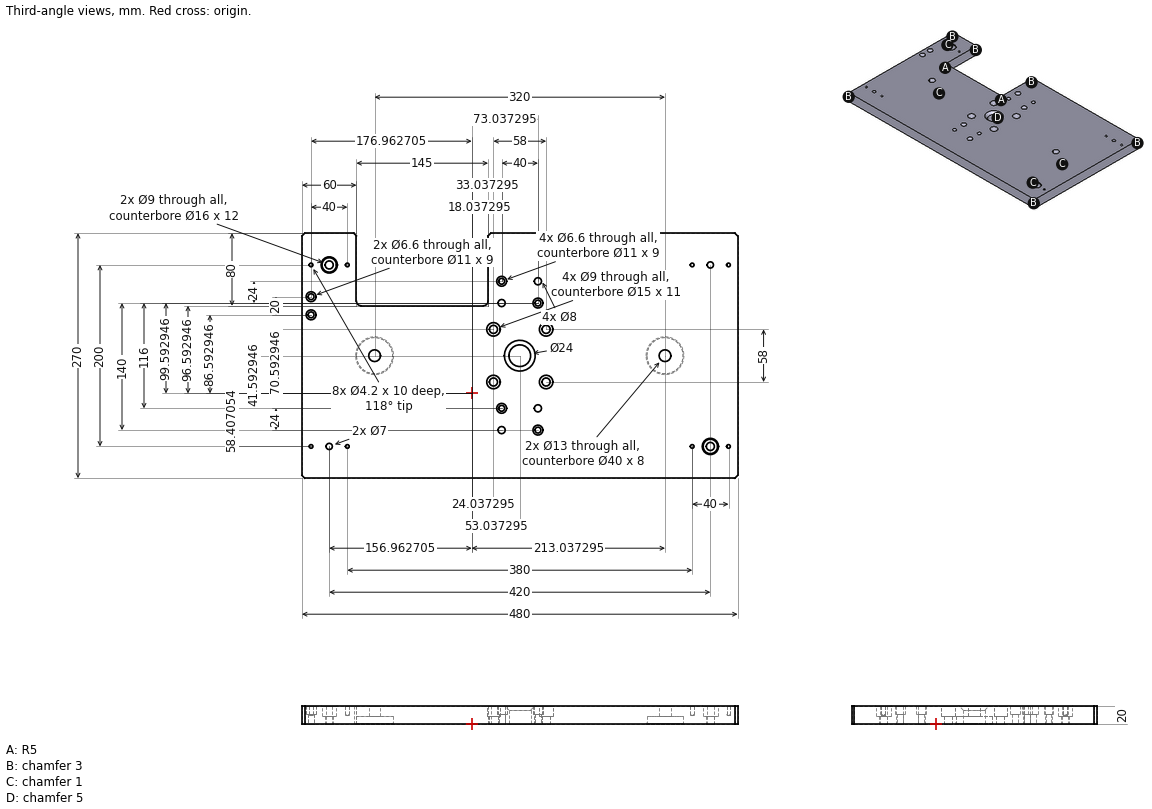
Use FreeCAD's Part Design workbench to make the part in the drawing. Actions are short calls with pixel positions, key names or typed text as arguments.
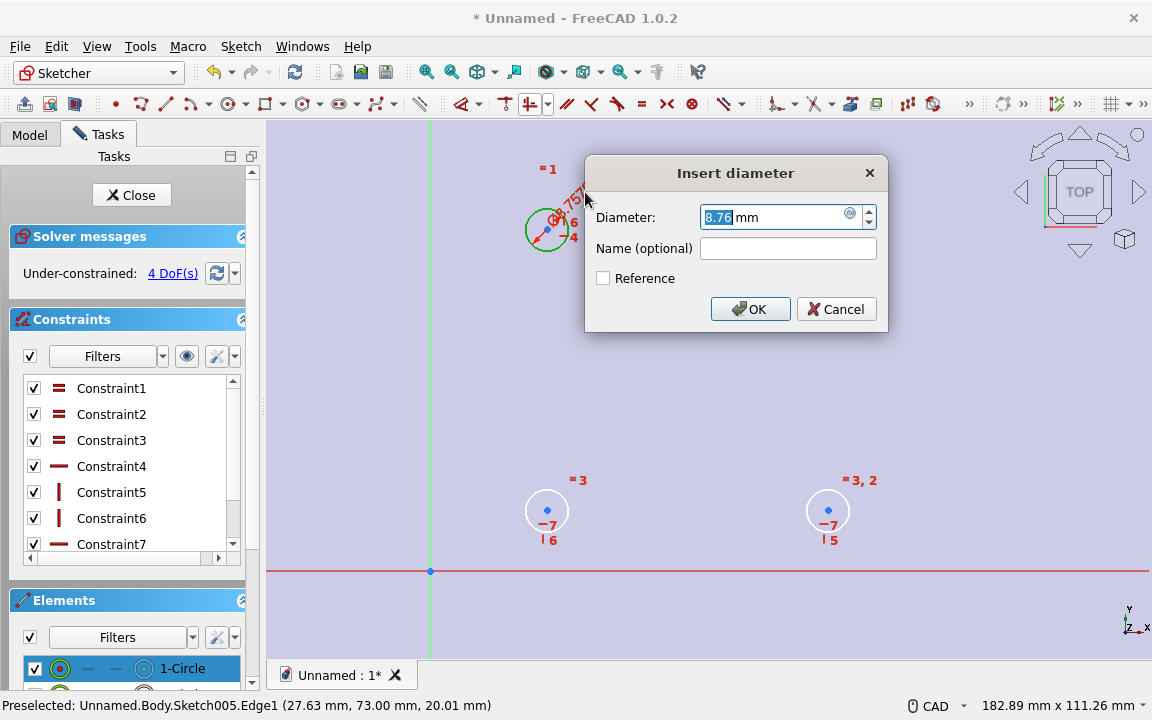
text(9)
key(Return)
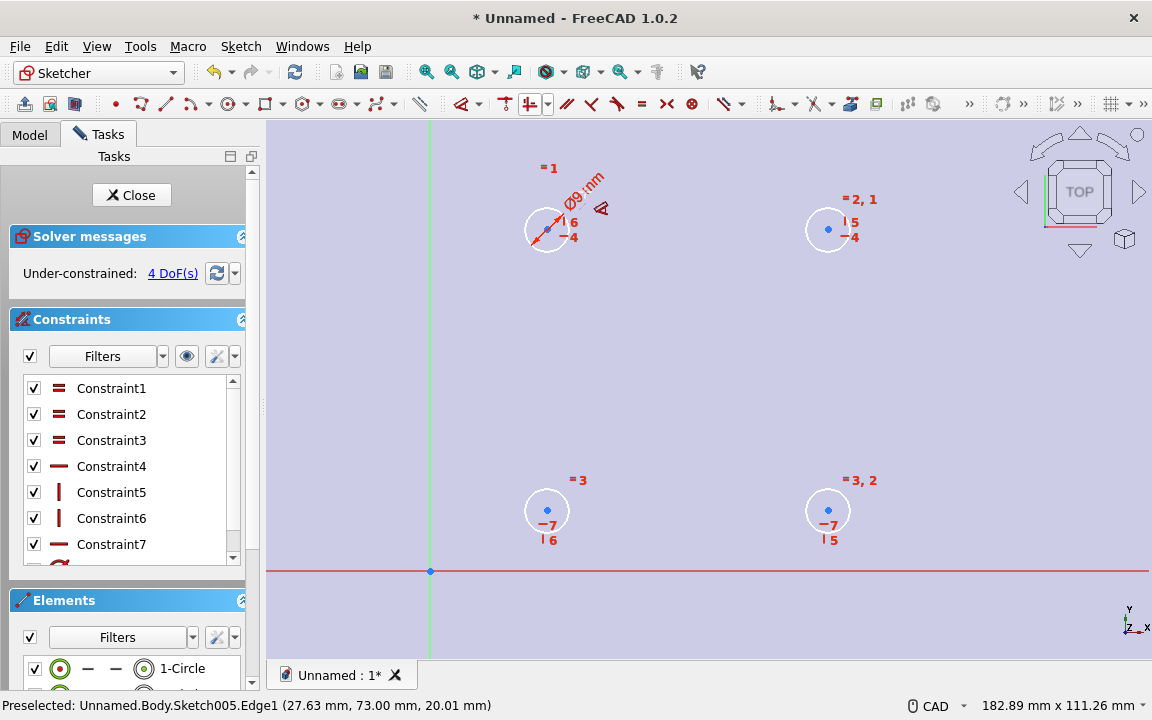
click(547, 230)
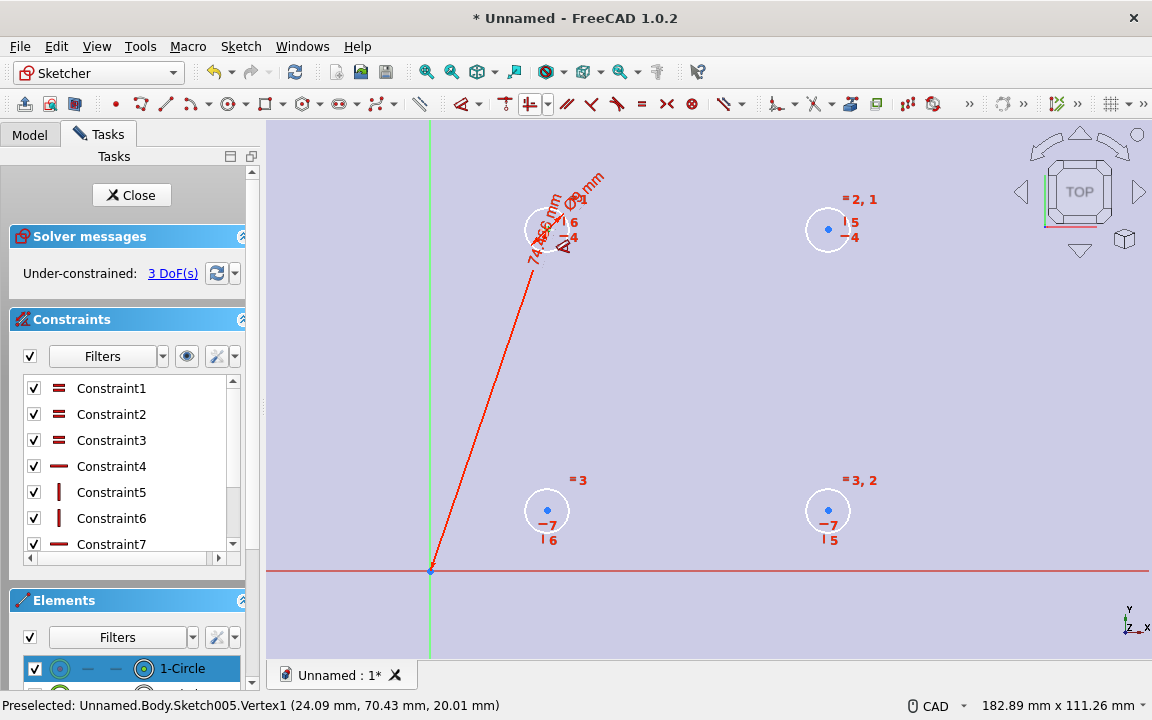
click(828, 230)
click(687, 196)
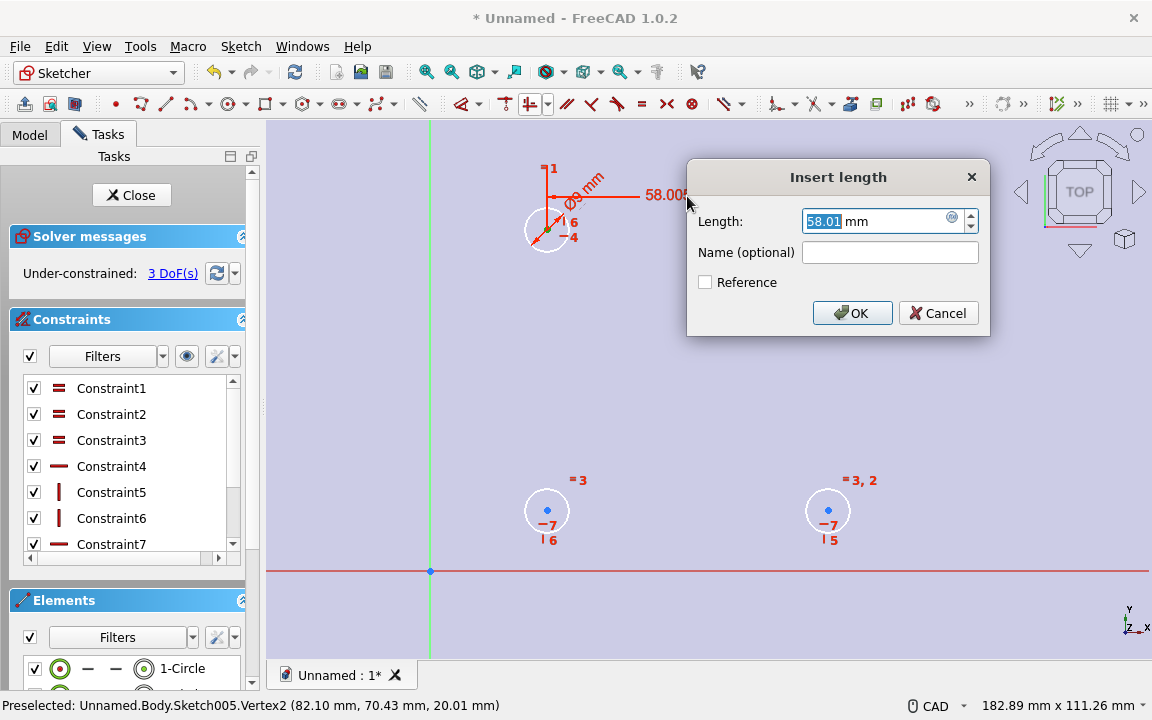
text(58)
key(Return)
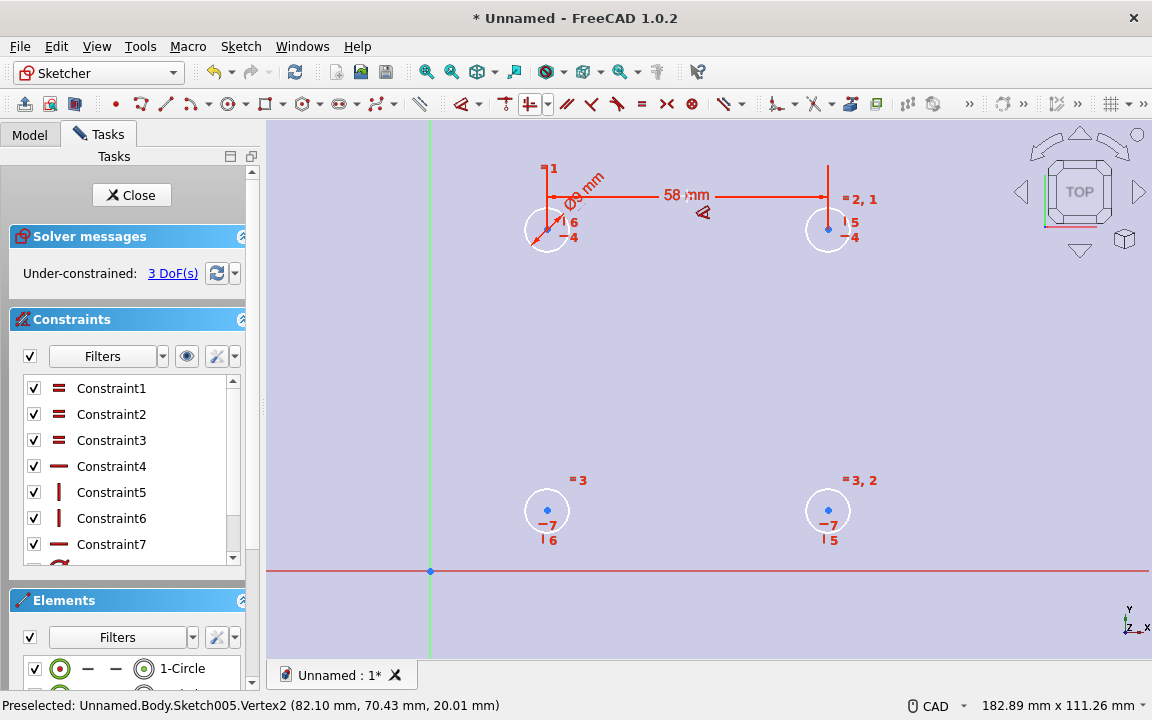
click(828, 230)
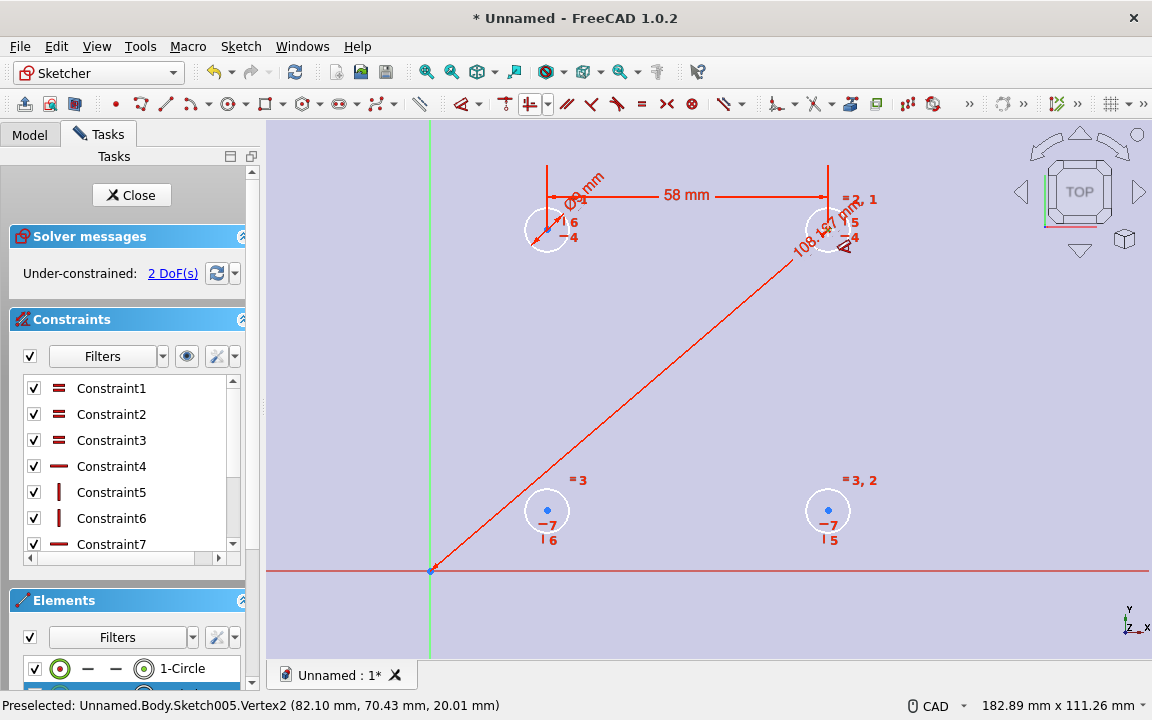
click(828, 511)
click(862, 371)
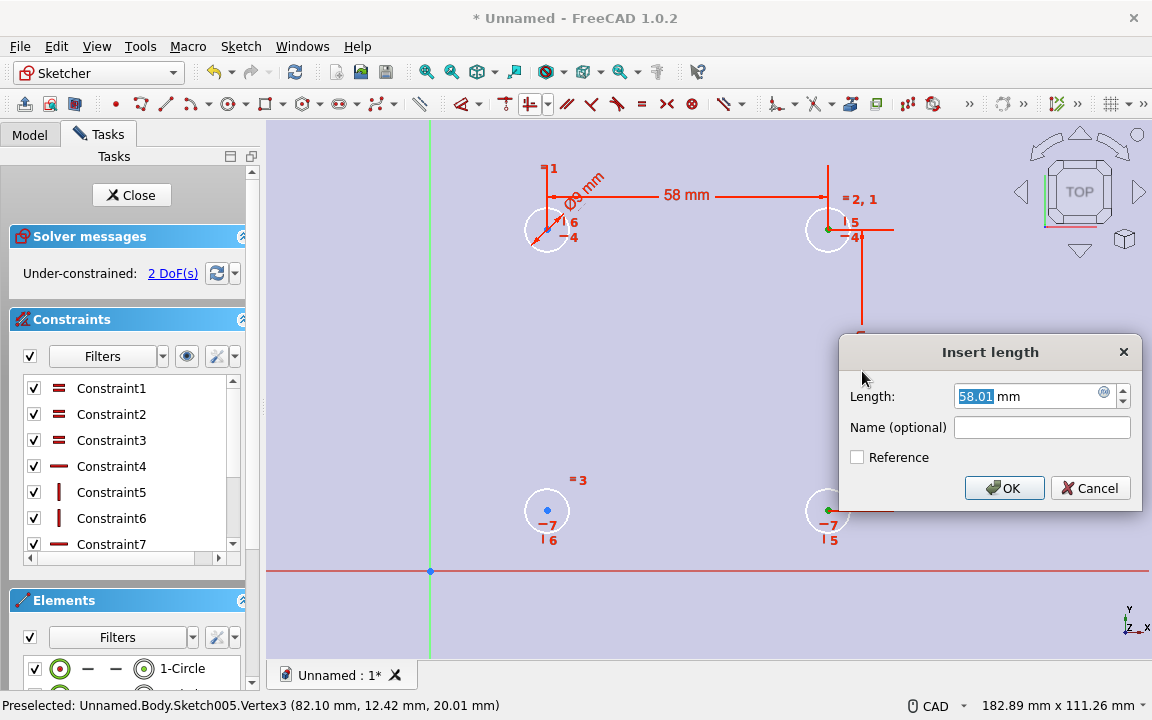
text(58)
key(Return)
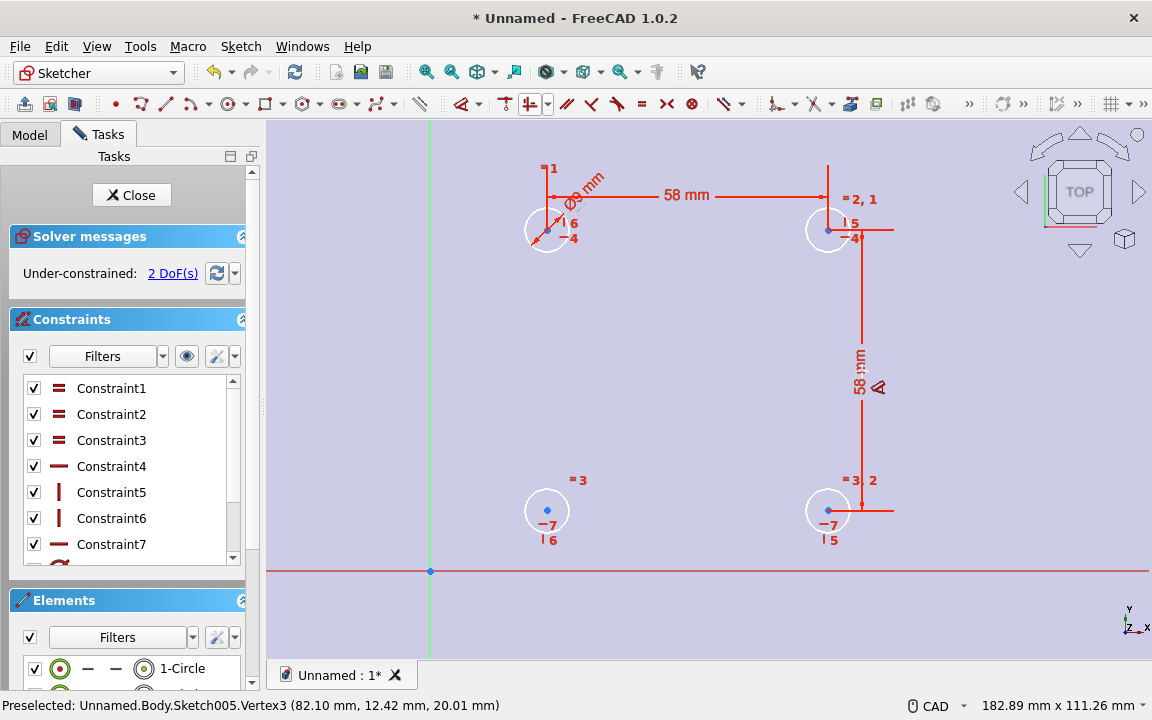
click(547, 230)
click(489, 605)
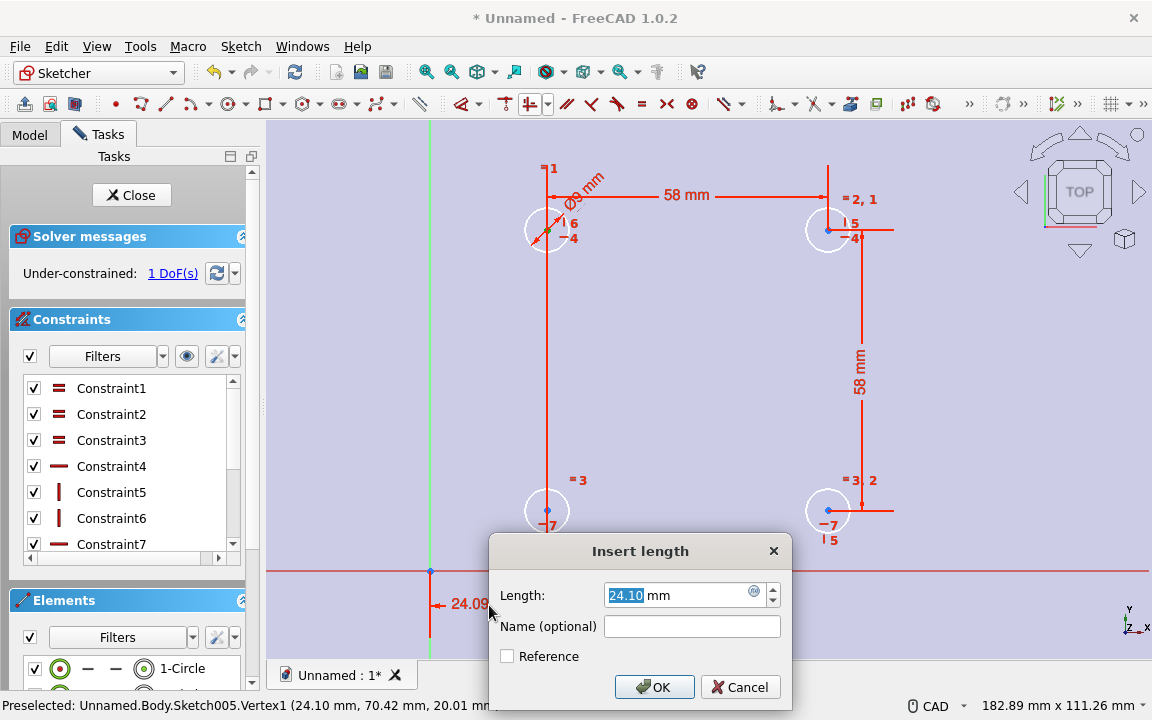
text(24.037295)
key(Return)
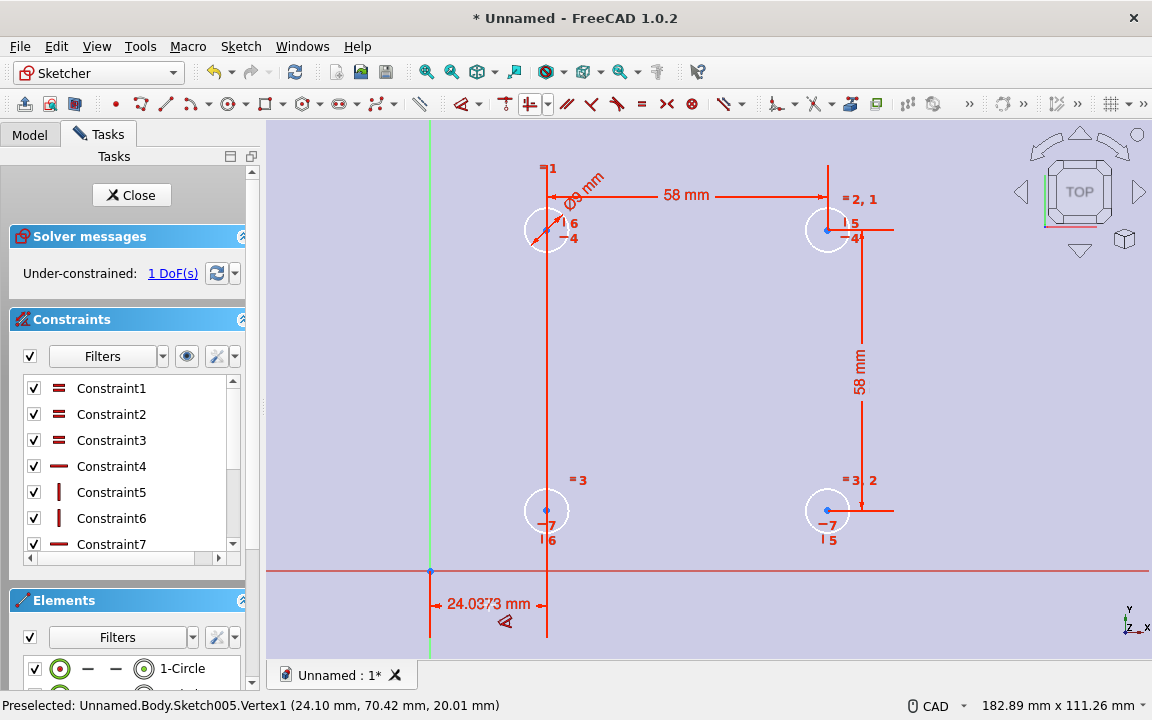
click(547, 230)
click(396, 401)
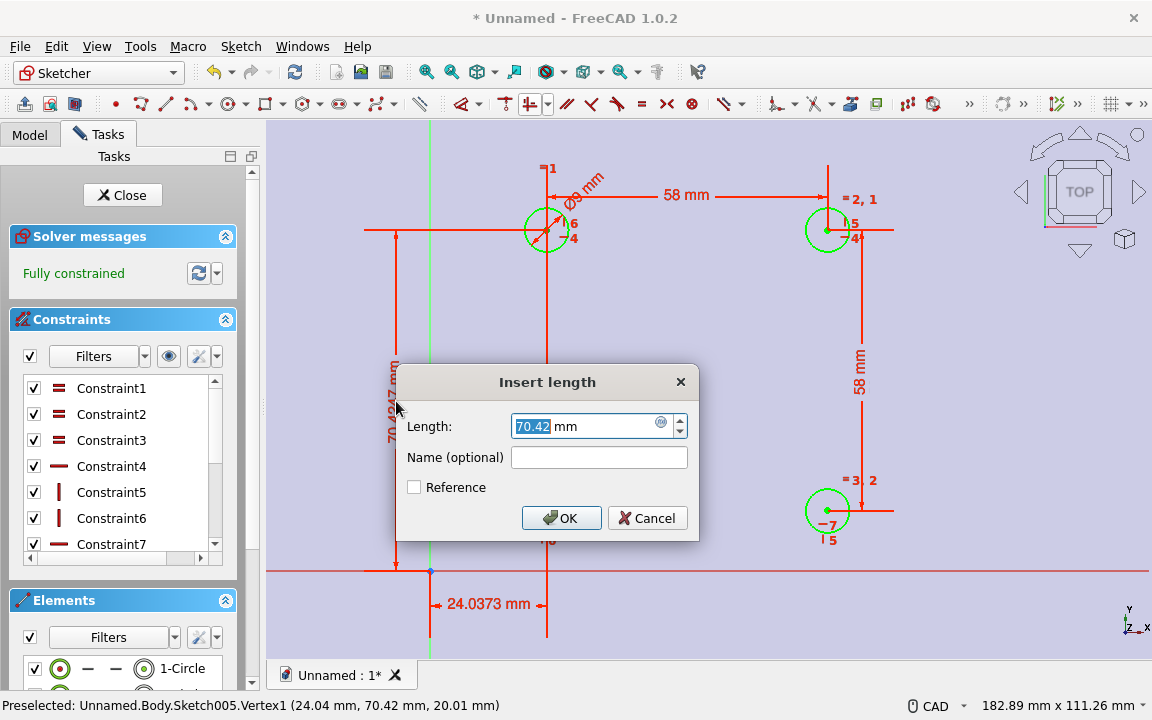
text(70.592946)
key(Return)
key(Escape)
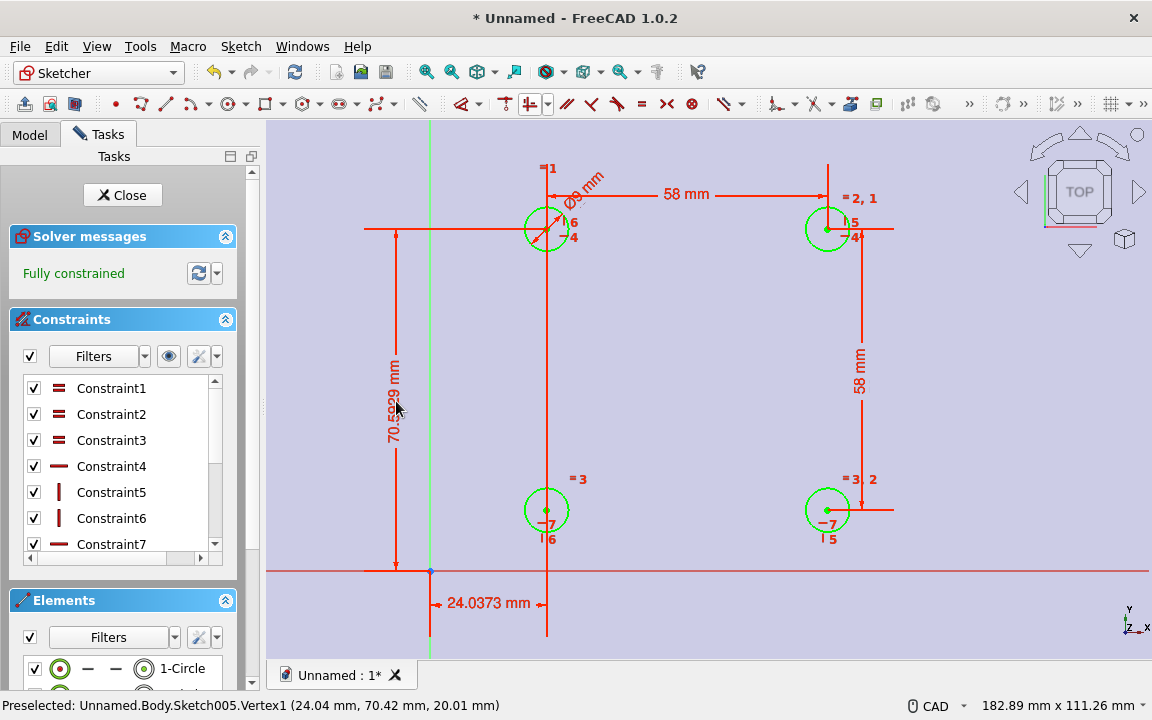
click(123, 195)